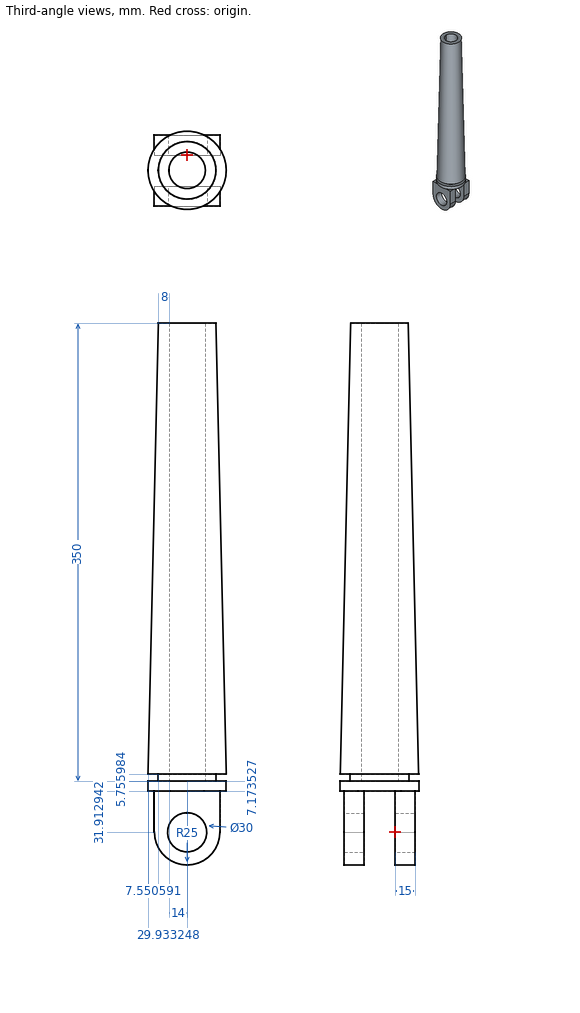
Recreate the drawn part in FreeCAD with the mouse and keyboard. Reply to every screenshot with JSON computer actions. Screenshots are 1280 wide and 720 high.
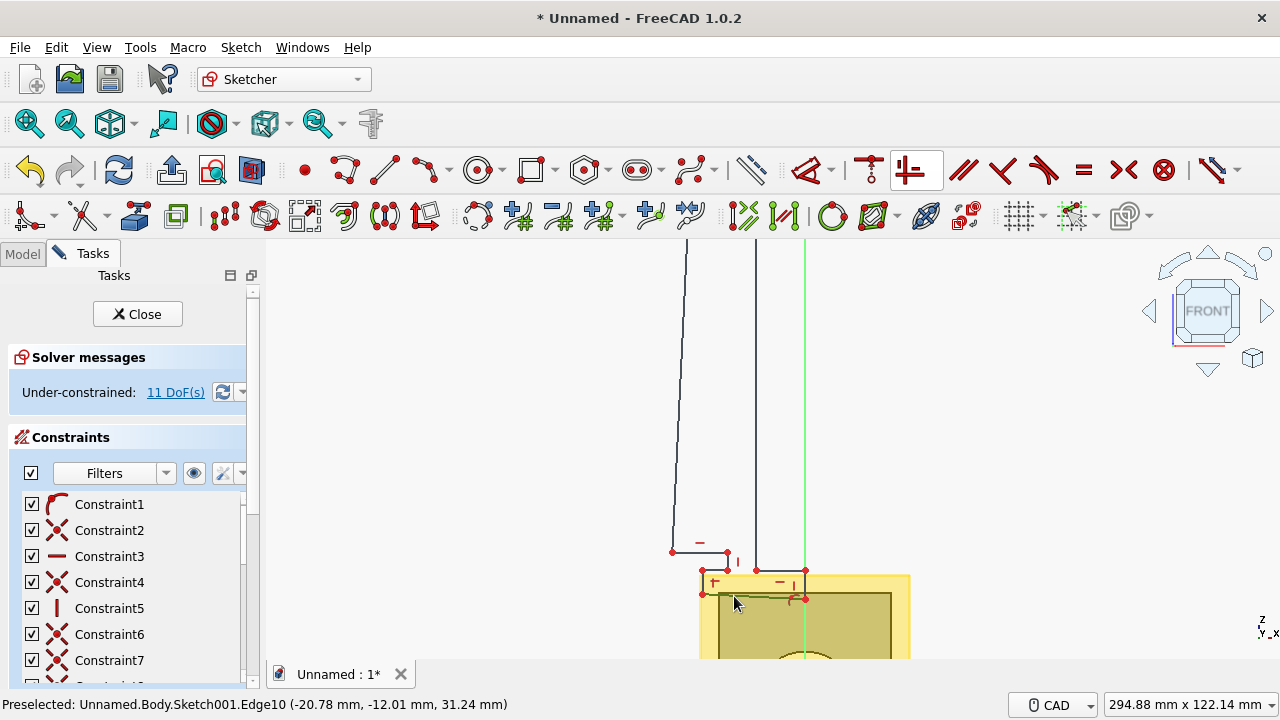
{"action": "left_click", "coordinate": [938, 170]}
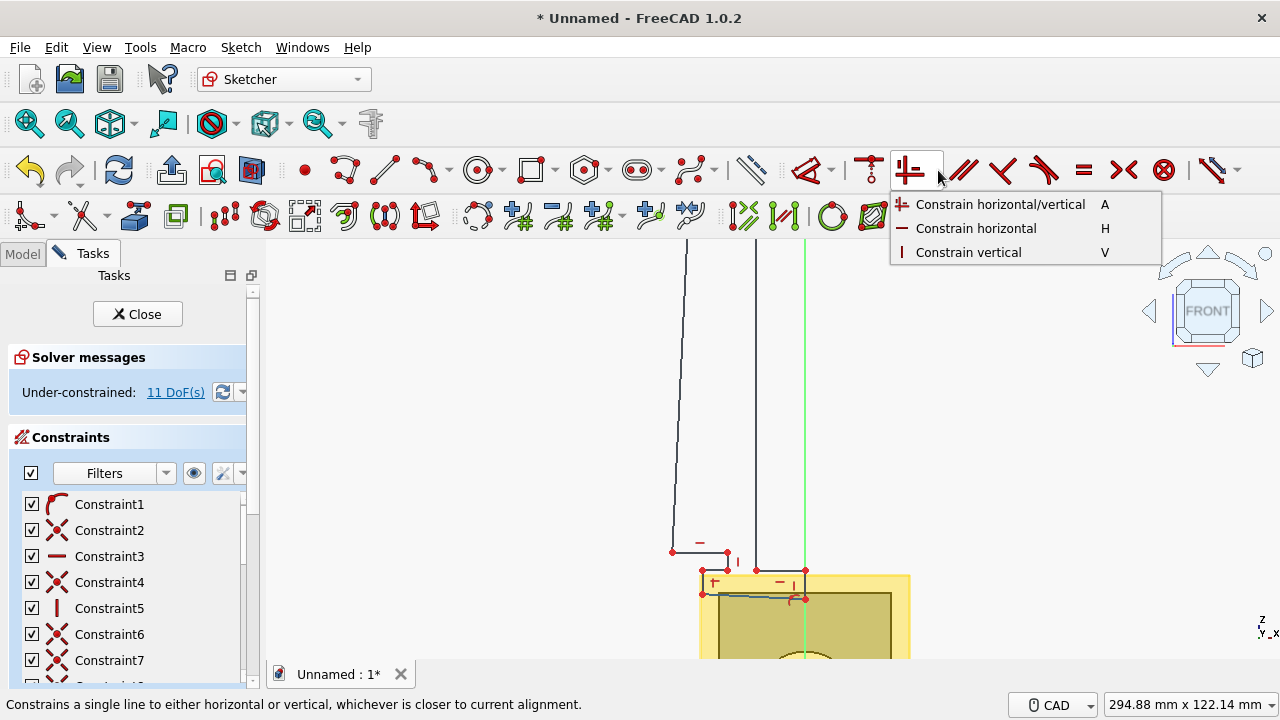
{"action": "left_click", "coordinate": [1026, 228]}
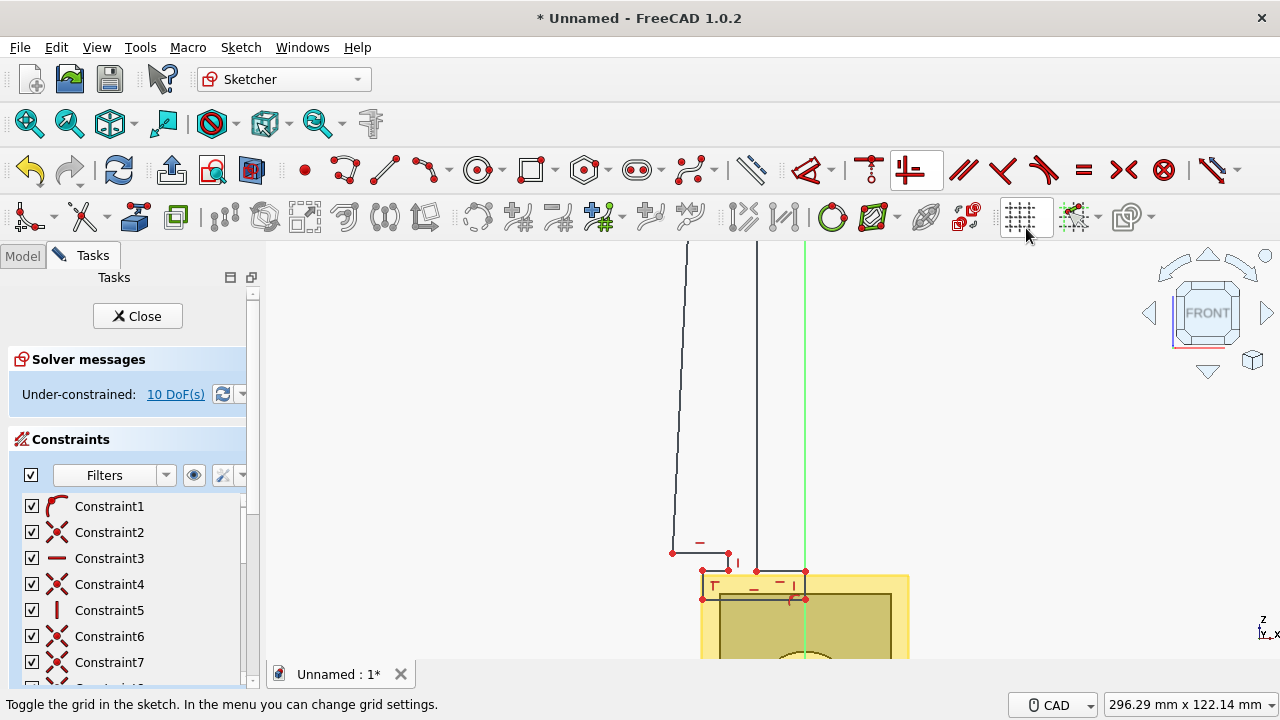
{"action": "left_click", "coordinate": [806, 170]}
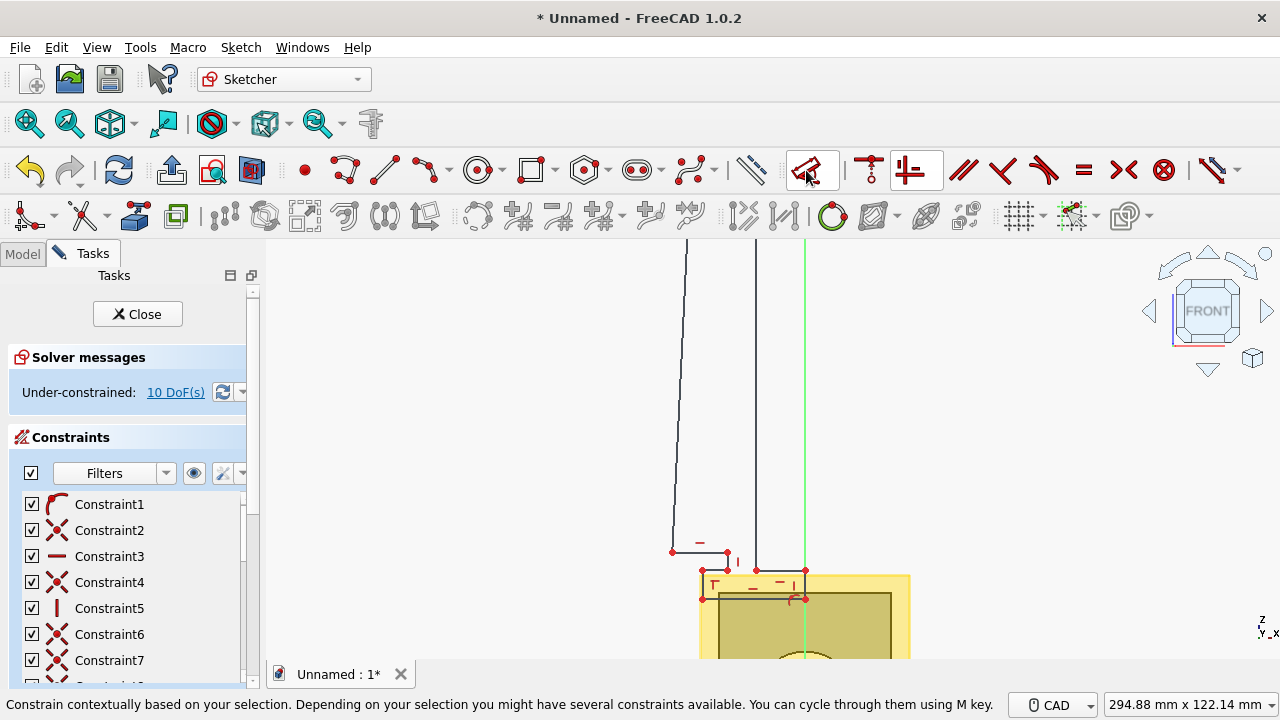
{"action": "scroll", "coordinate": [692, 554], "scroll_direction": "down", "scroll_amount": 8}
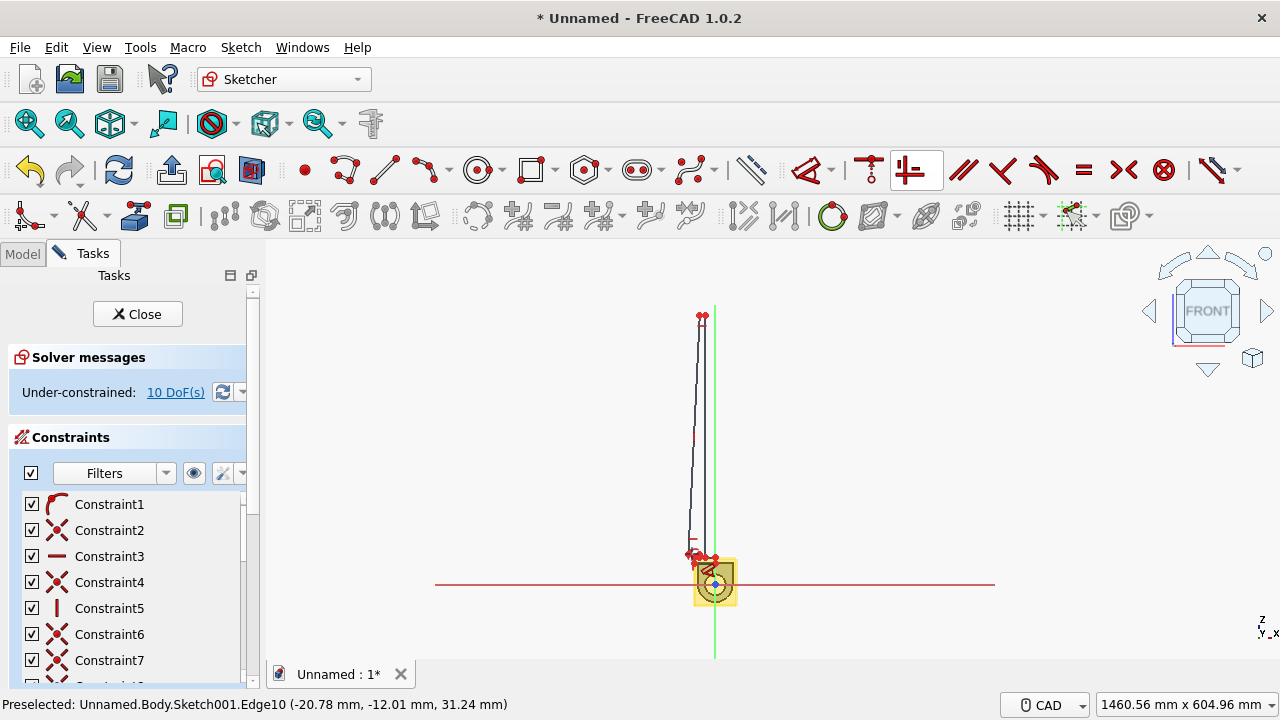
{"action": "scroll", "coordinate": [703, 315], "scroll_direction": "up", "scroll_amount": 10}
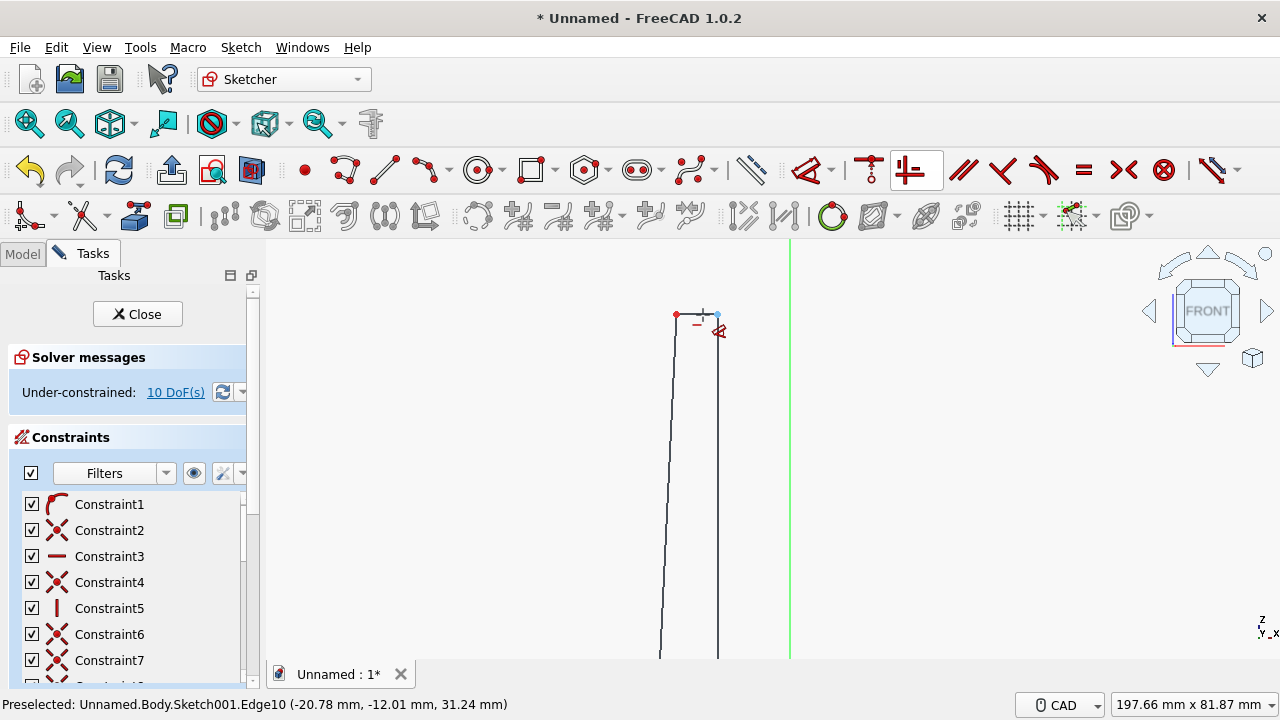
{"action": "left_click", "coordinate": [701, 314]}
{"action": "left_click", "coordinate": [697, 280]}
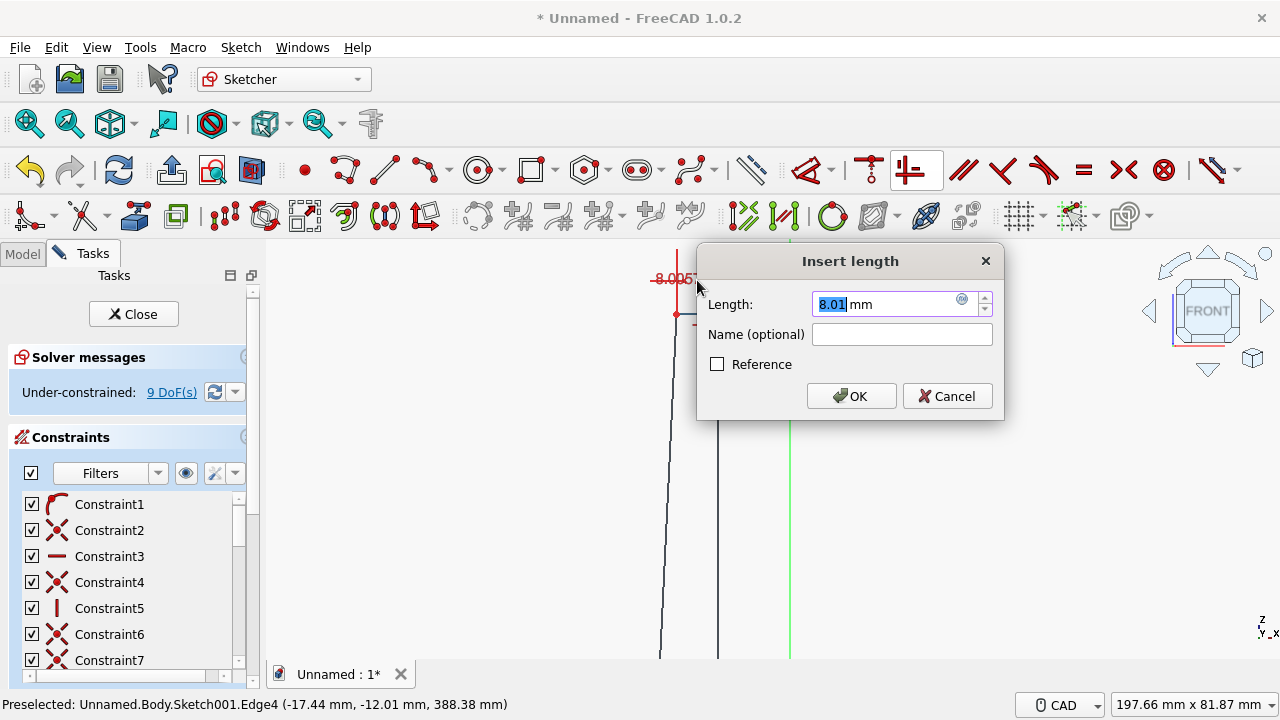
{"action": "type", "text": "8"}
{"action": "key", "text": "Return"}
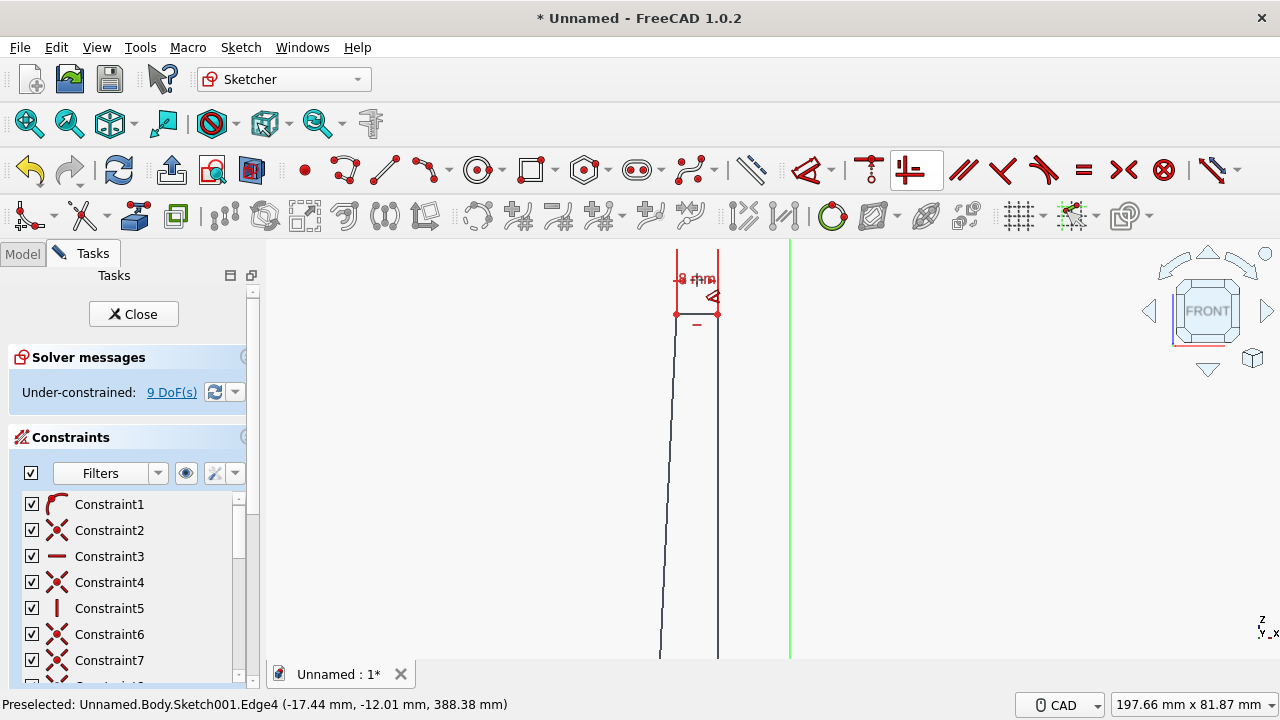
{"action": "scroll", "coordinate": [703, 314], "scroll_direction": "down", "scroll_amount": 10}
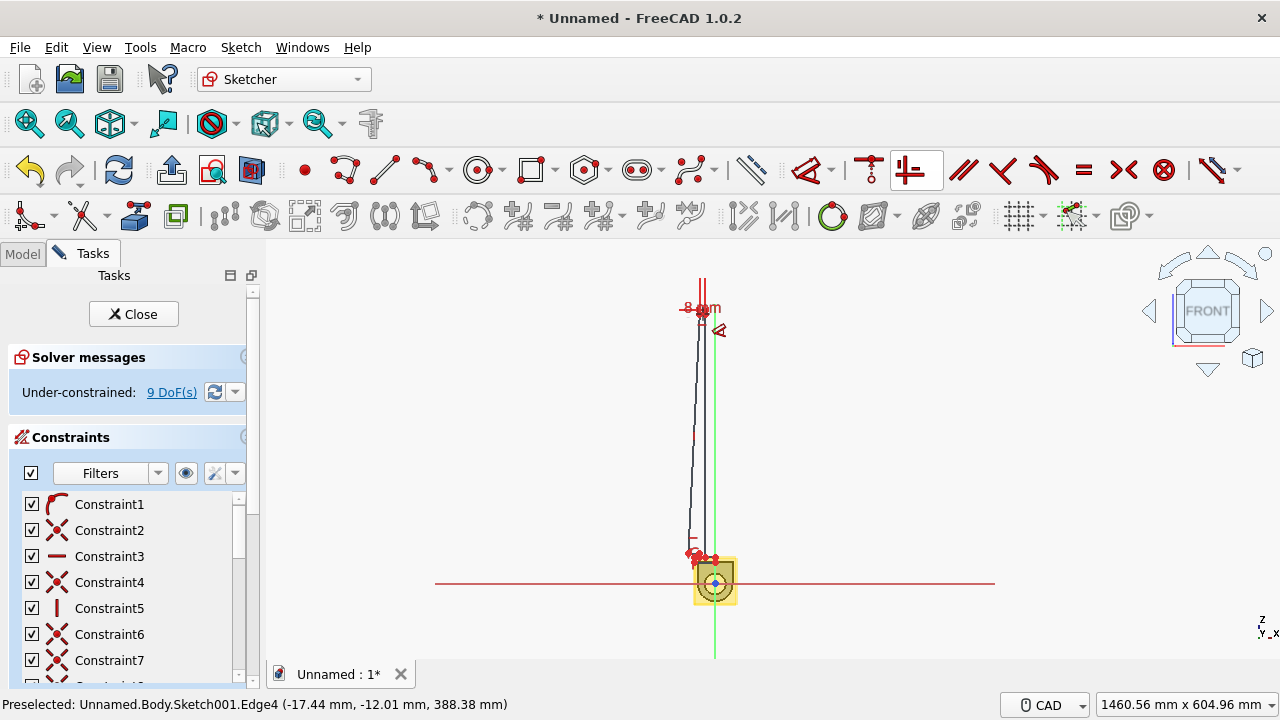
{"action": "scroll", "coordinate": [712, 557], "scroll_direction": "up", "scroll_amount": 8}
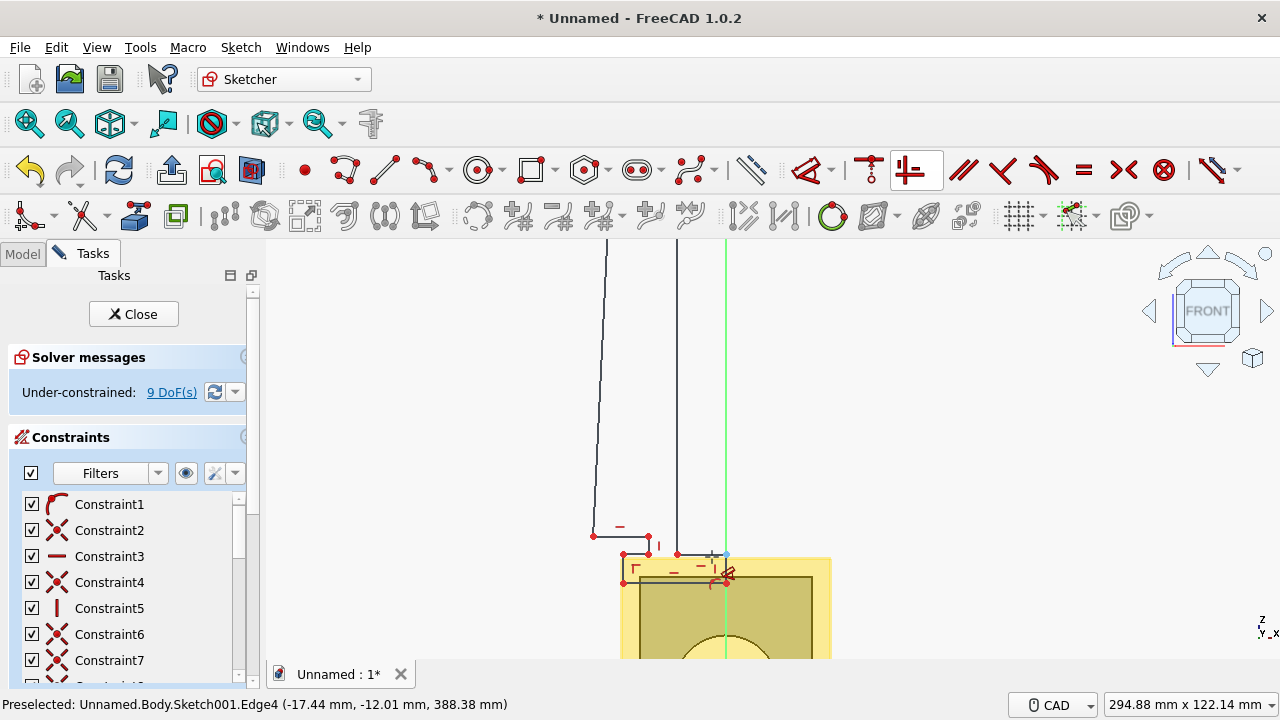
{"action": "left_click", "coordinate": [712, 555]}
{"action": "left_click", "coordinate": [702, 521]}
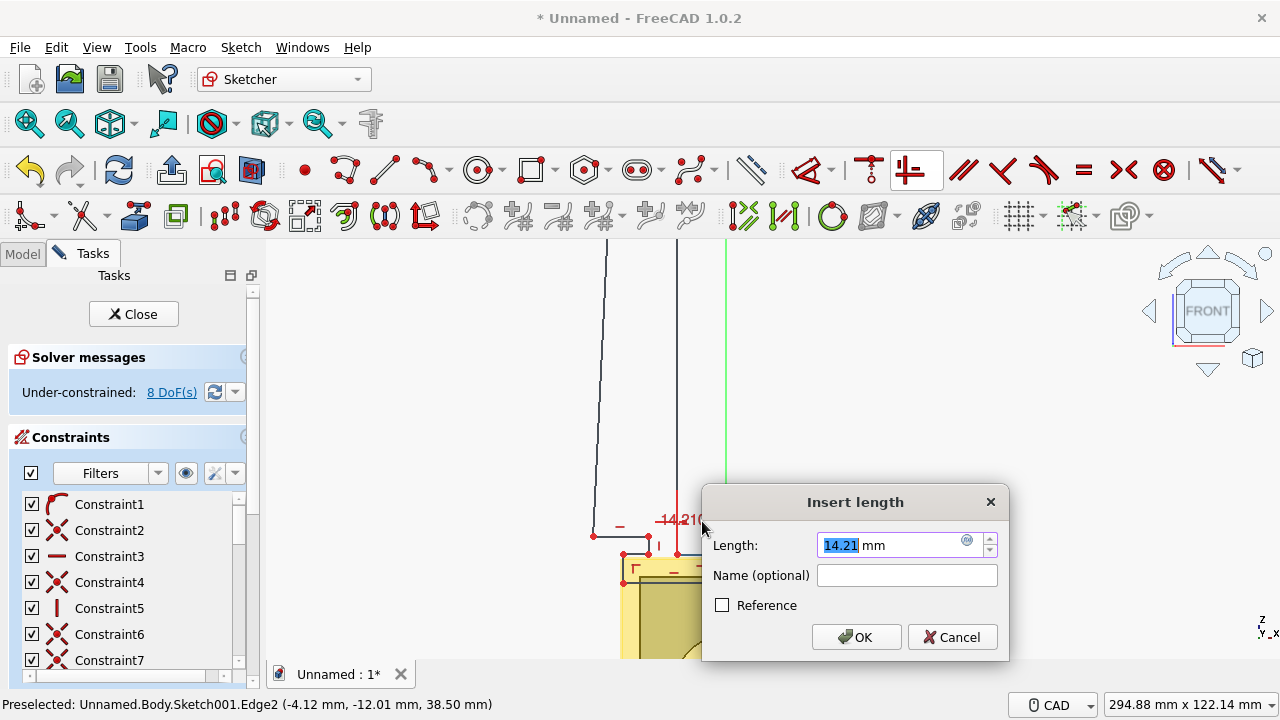
{"action": "type", "text": "14"}
{"action": "key", "text": "Return"}